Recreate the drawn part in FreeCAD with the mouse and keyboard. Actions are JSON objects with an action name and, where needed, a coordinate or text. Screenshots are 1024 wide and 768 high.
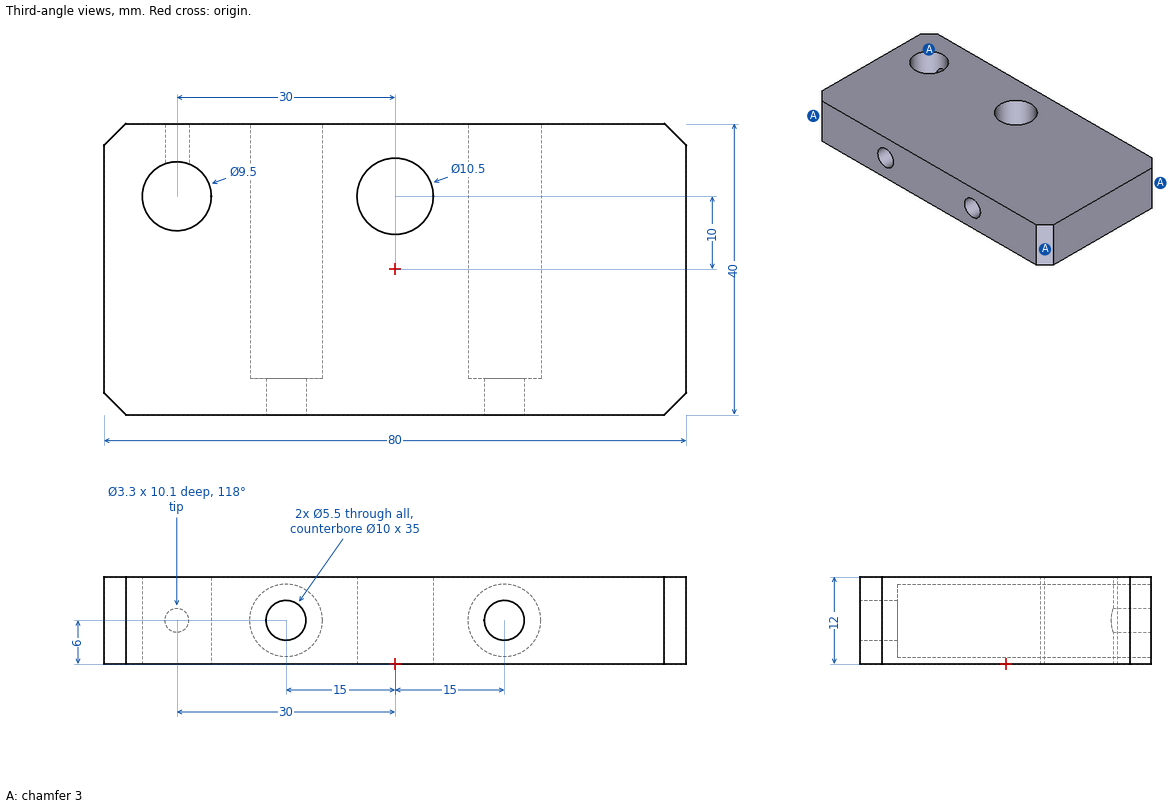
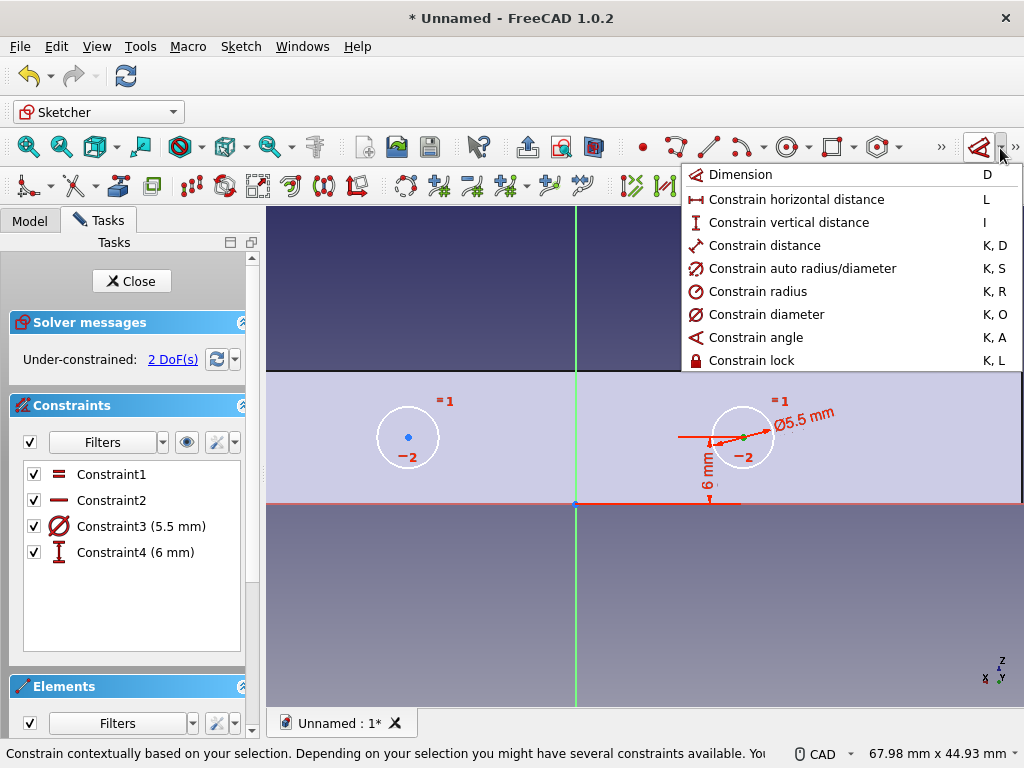
{"action": "left_click", "coordinate": [852, 200]}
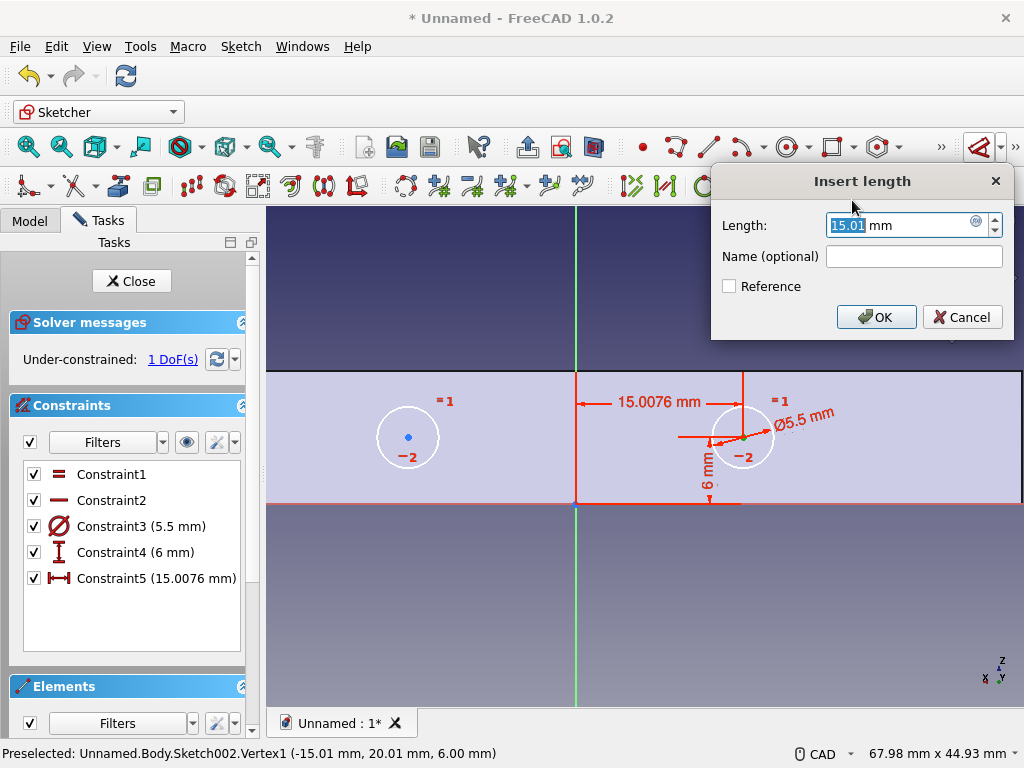
{"action": "type", "text": "15"}
{"action": "key", "text": "Return"}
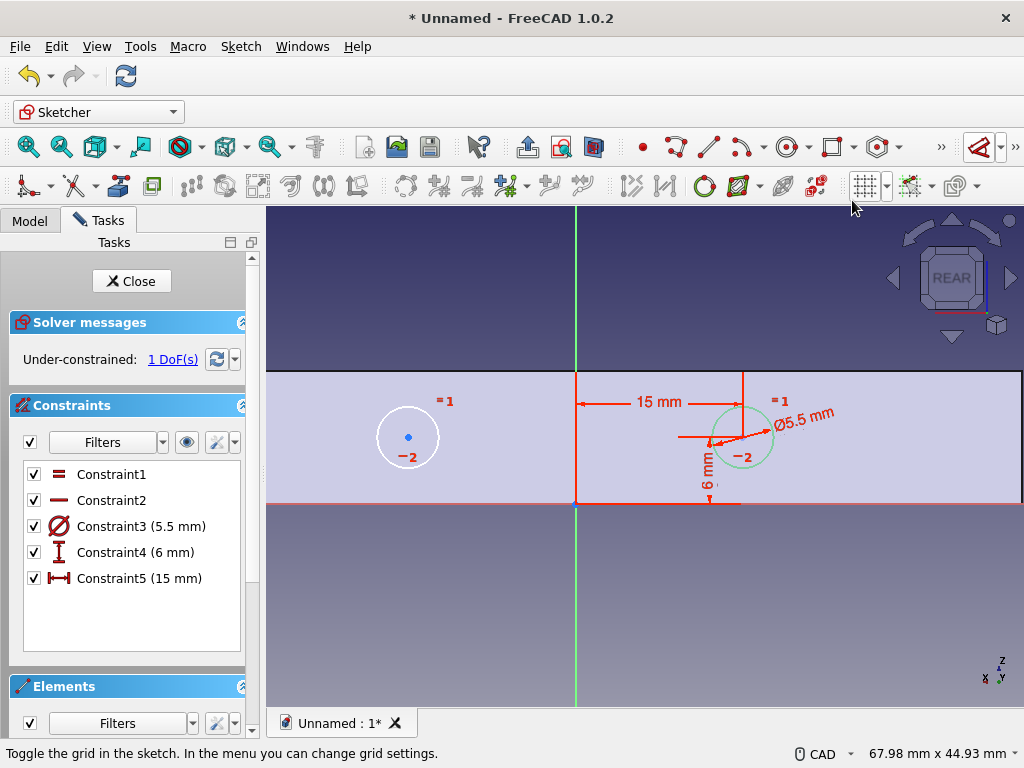
{"action": "left_click", "coordinate": [408, 437]}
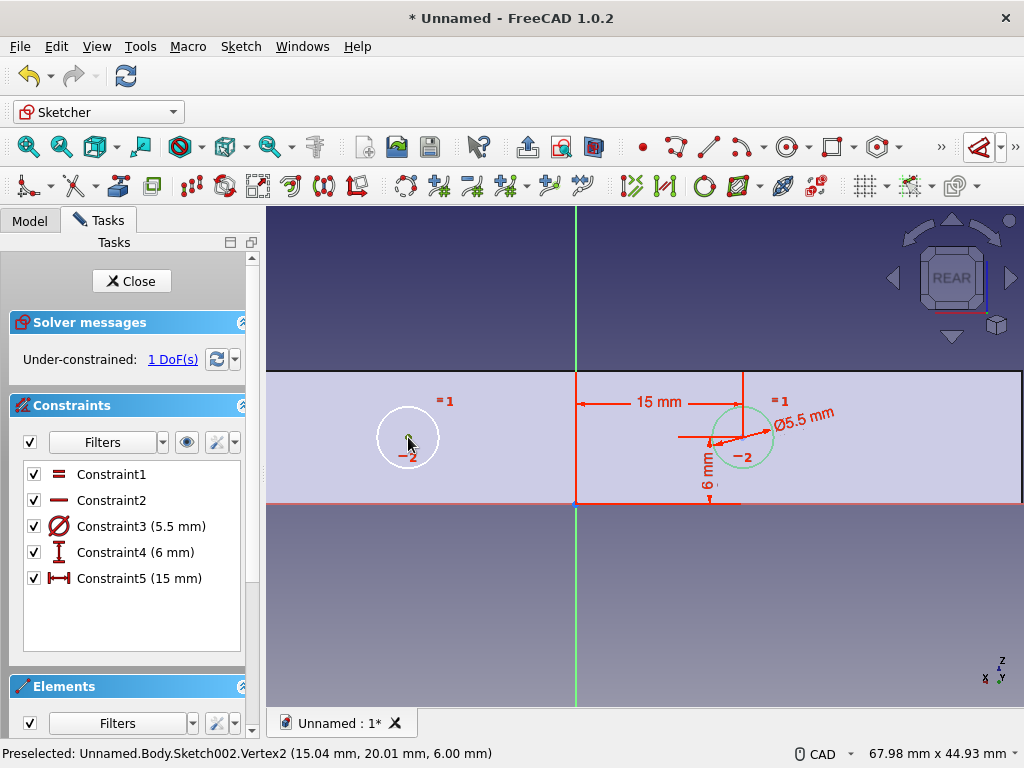
{"action": "key", "text": "l"}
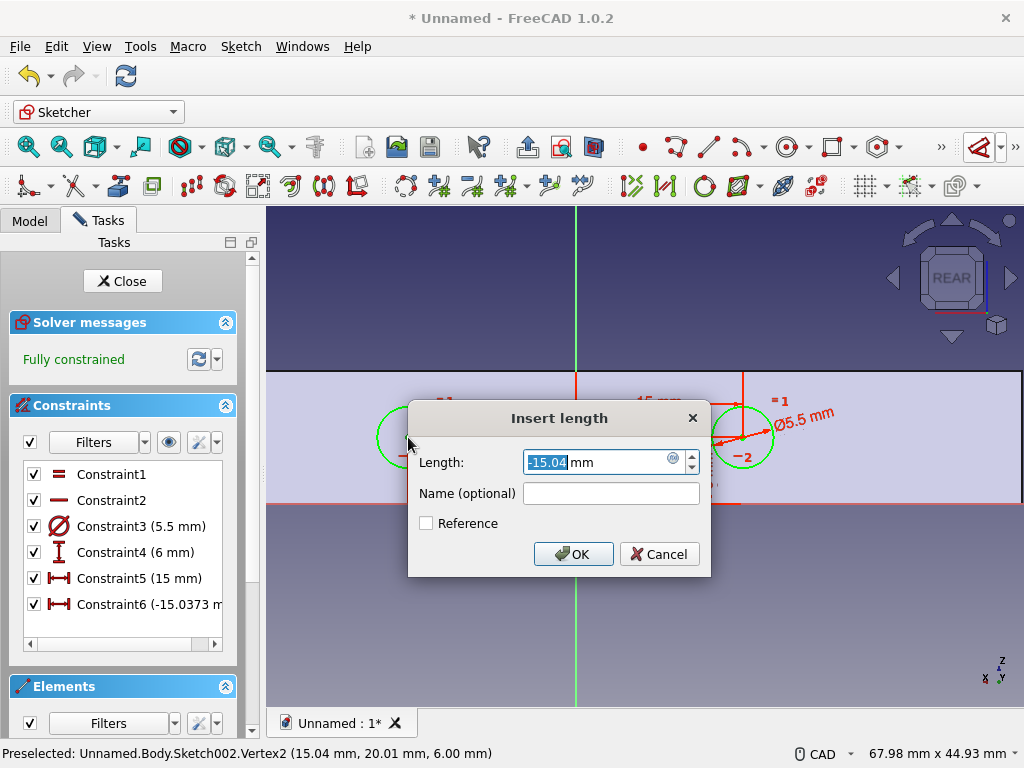
{"action": "type", "text": "-15"}
{"action": "key", "text": "Return"}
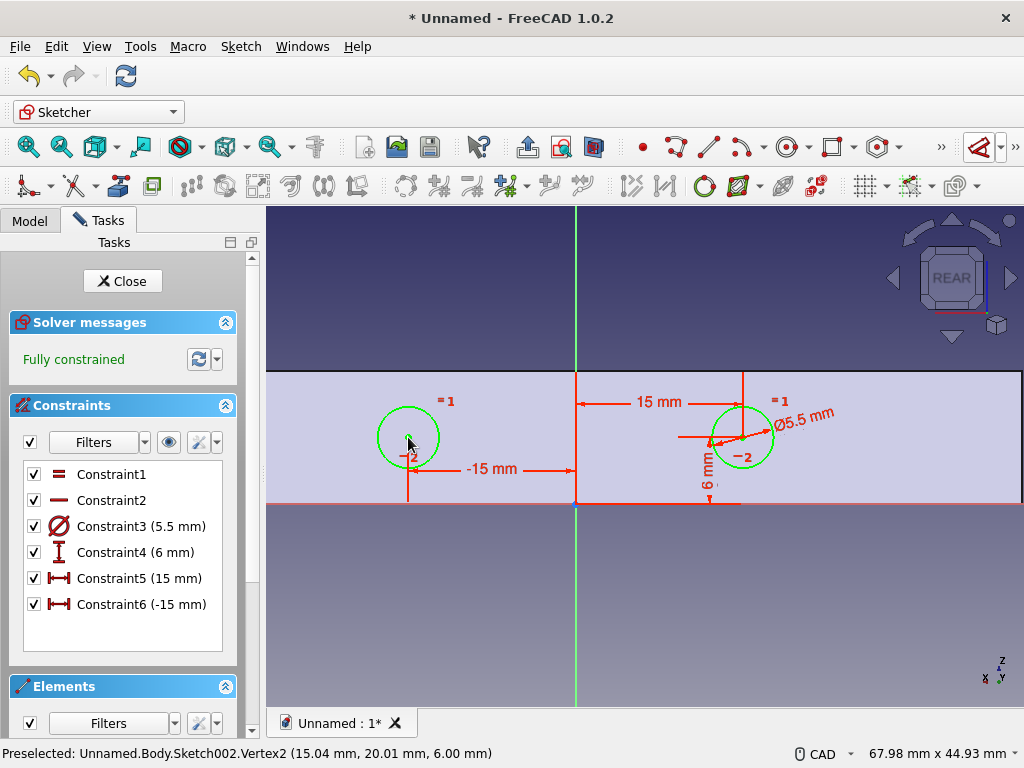
{"action": "left_click", "coordinate": [123, 281]}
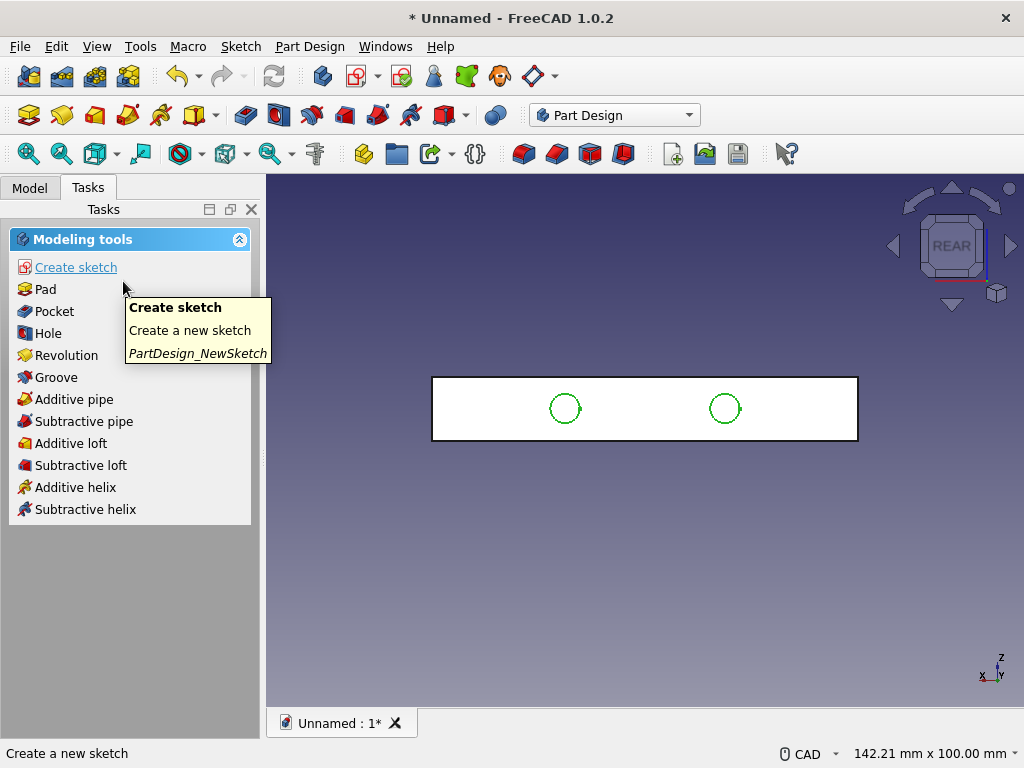
{"action": "left_click", "coordinate": [279, 116]}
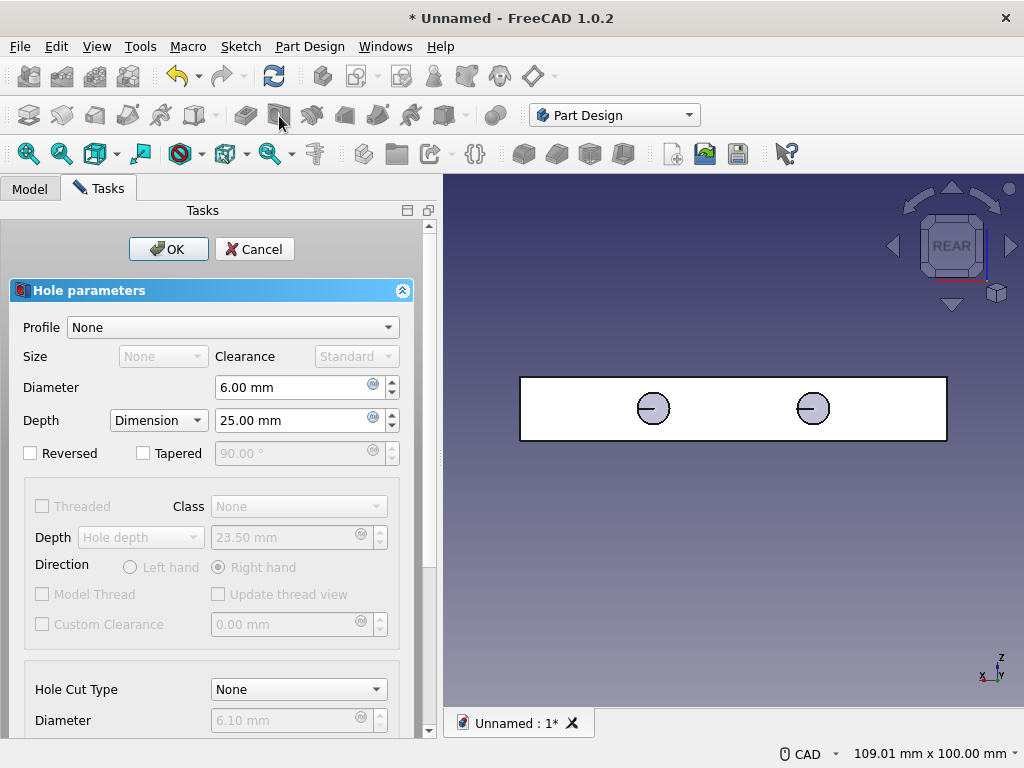
{"action": "triple_click", "coordinate": [300, 388]}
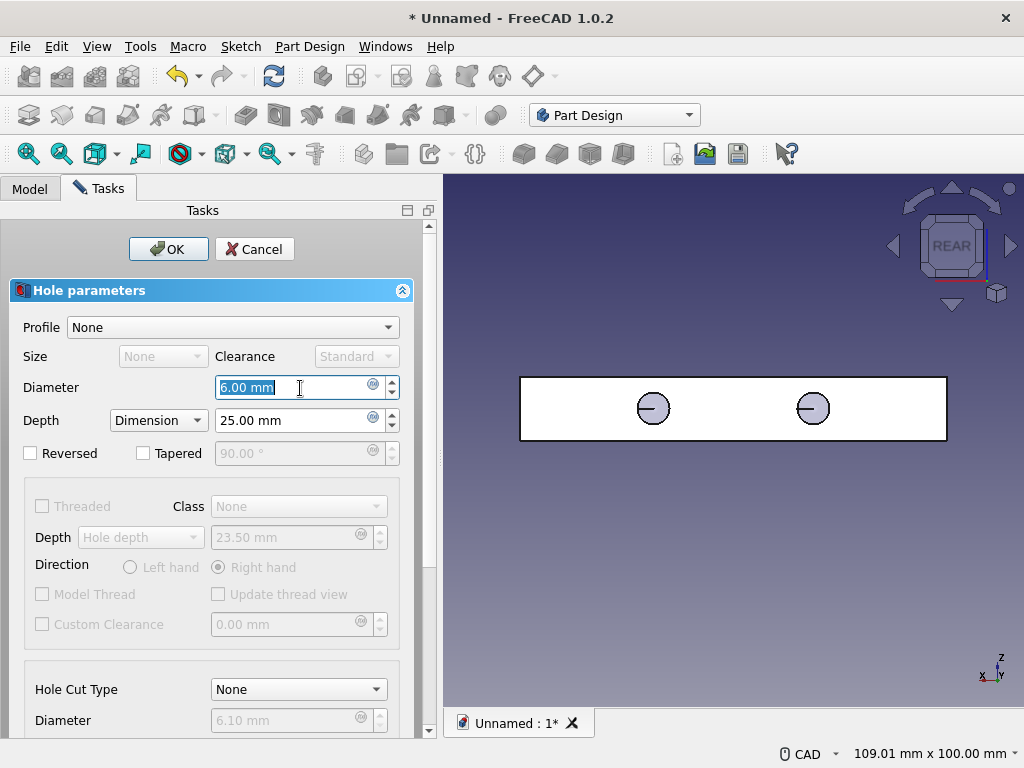
{"action": "type", "text": "5.5"}
{"action": "key", "text": "Tab"}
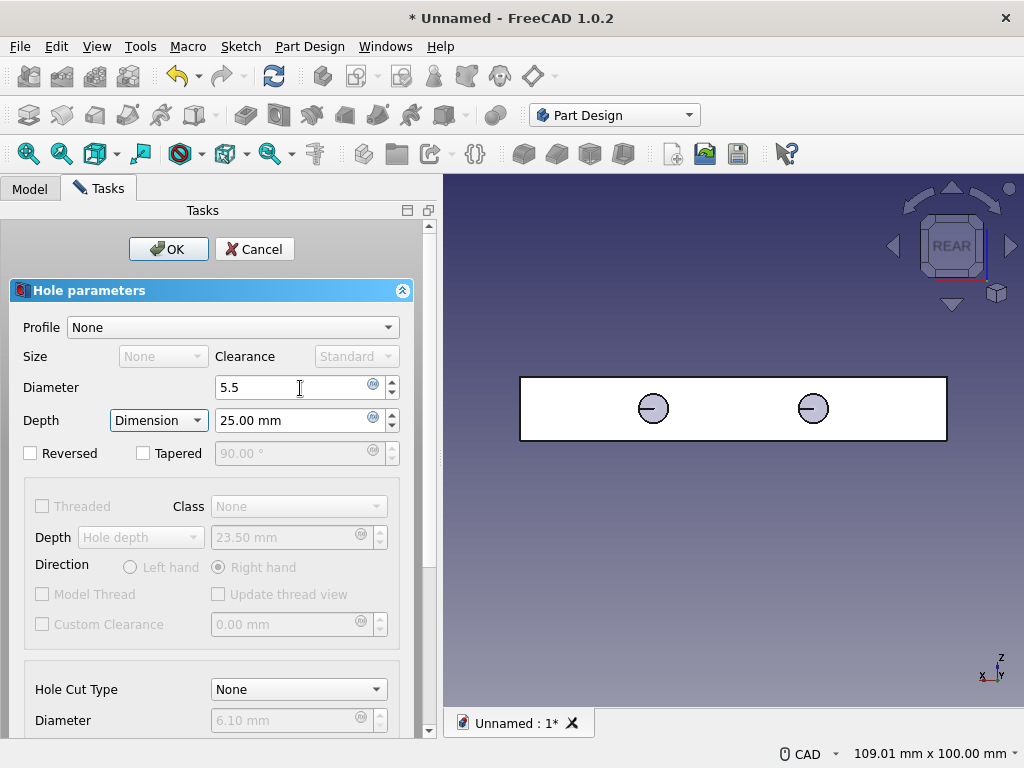
{"action": "left_click", "coordinate": [160, 420]}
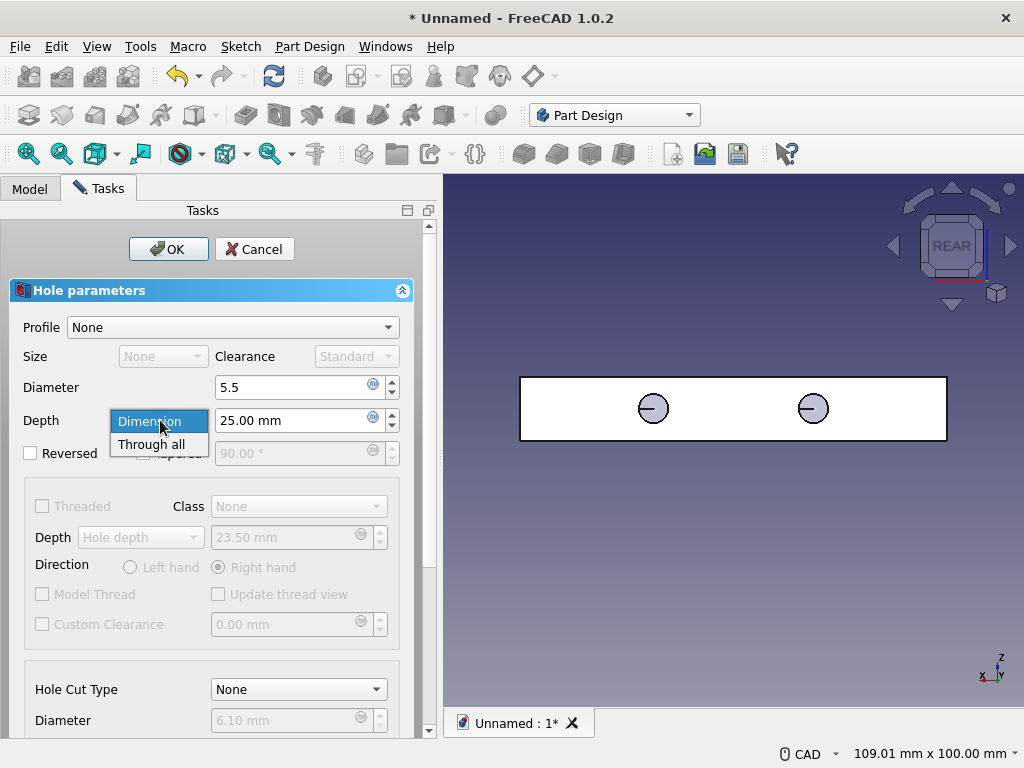
{"action": "left_click", "coordinate": [158, 444]}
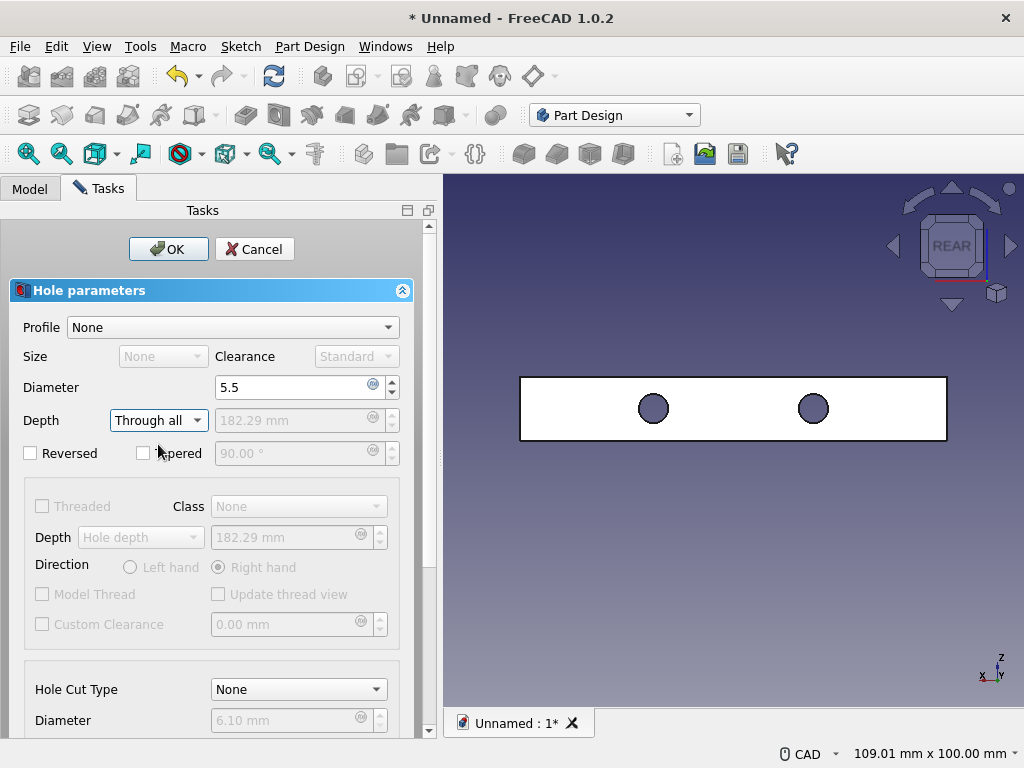
{"action": "left_click", "coordinate": [300, 690]}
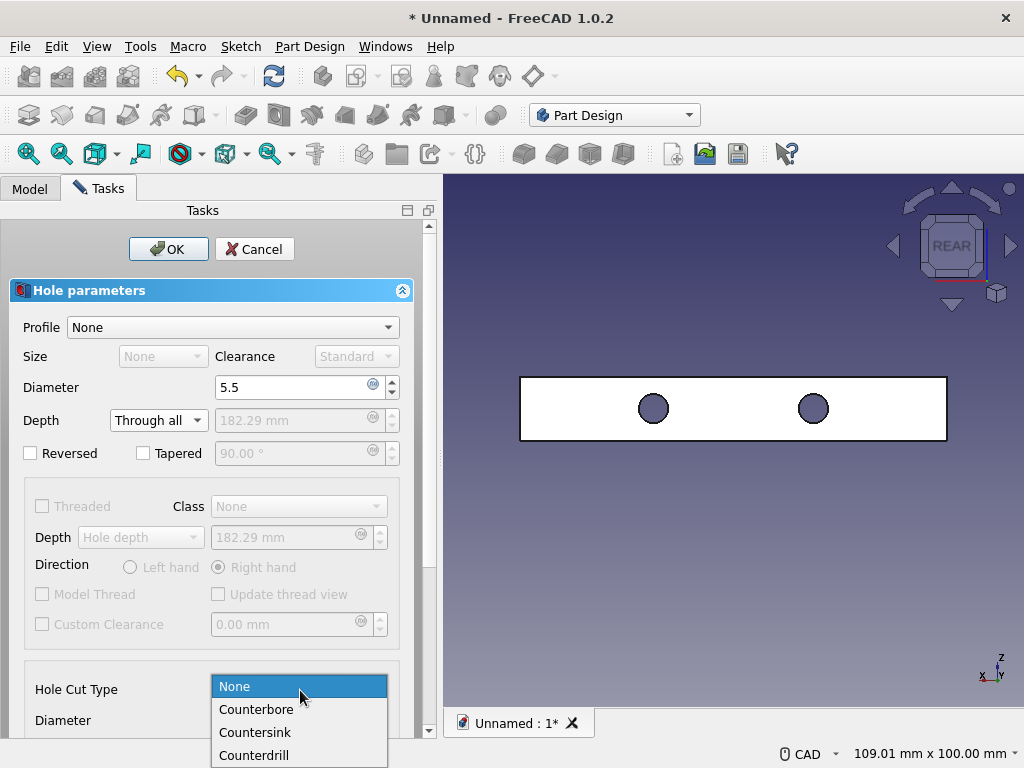
{"action": "left_click", "coordinate": [298, 710]}